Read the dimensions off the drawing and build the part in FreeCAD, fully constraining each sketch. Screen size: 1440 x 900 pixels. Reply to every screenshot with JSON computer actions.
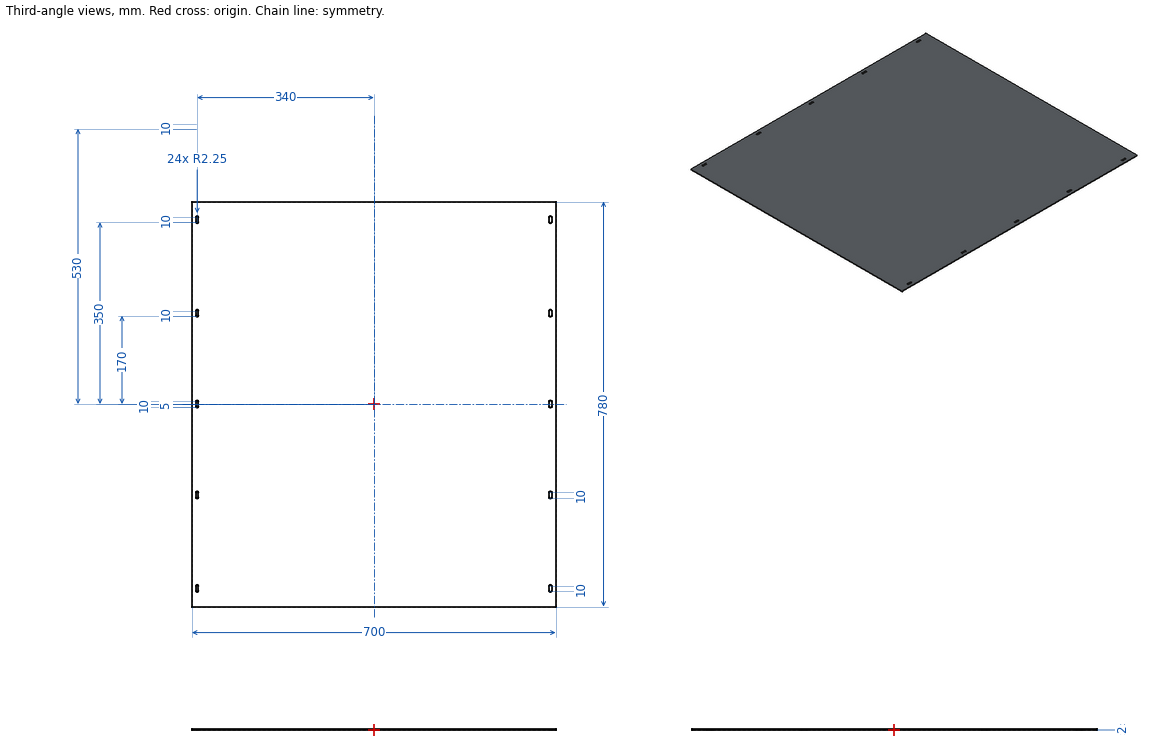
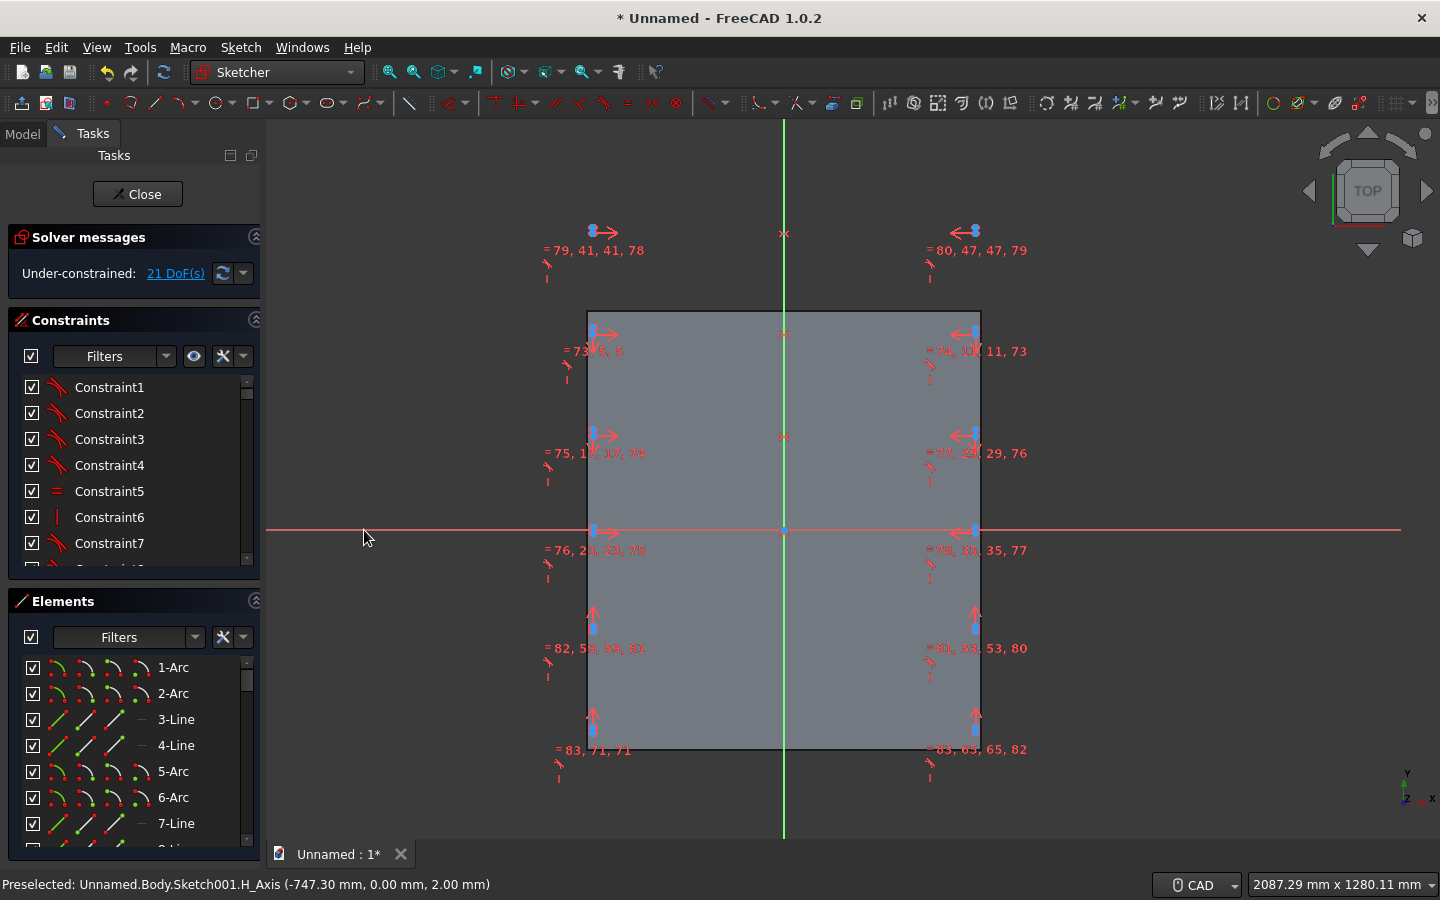
{"action": "key", "text": "d"}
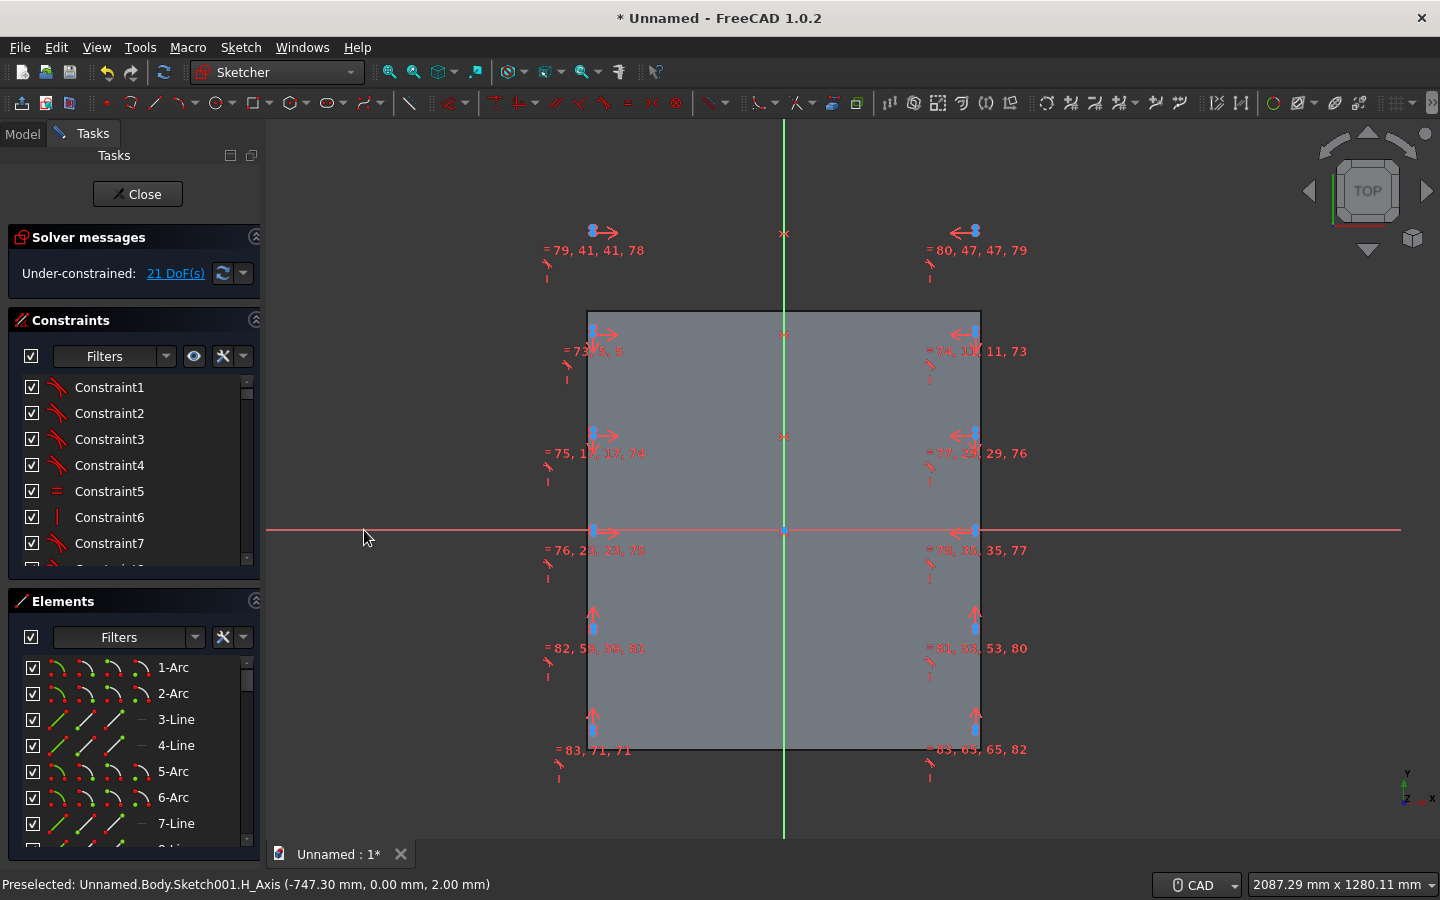
{"action": "scroll", "coordinate": [592, 331], "scroll_direction": "up", "scroll_amount": 10}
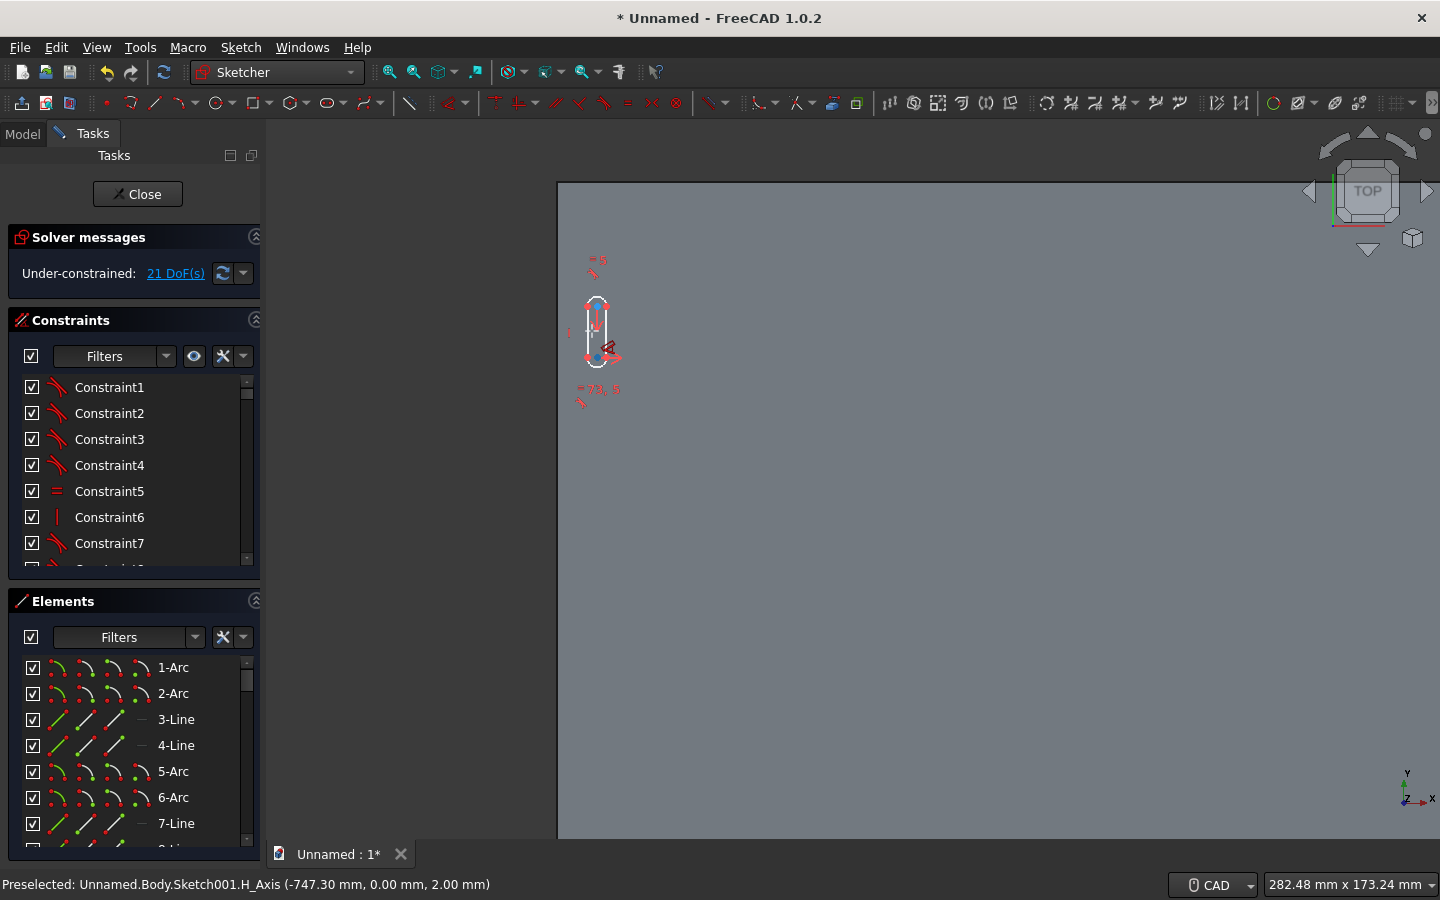
{"action": "left_click", "coordinate": [588, 327]}
{"action": "left_click", "coordinate": [554, 332]}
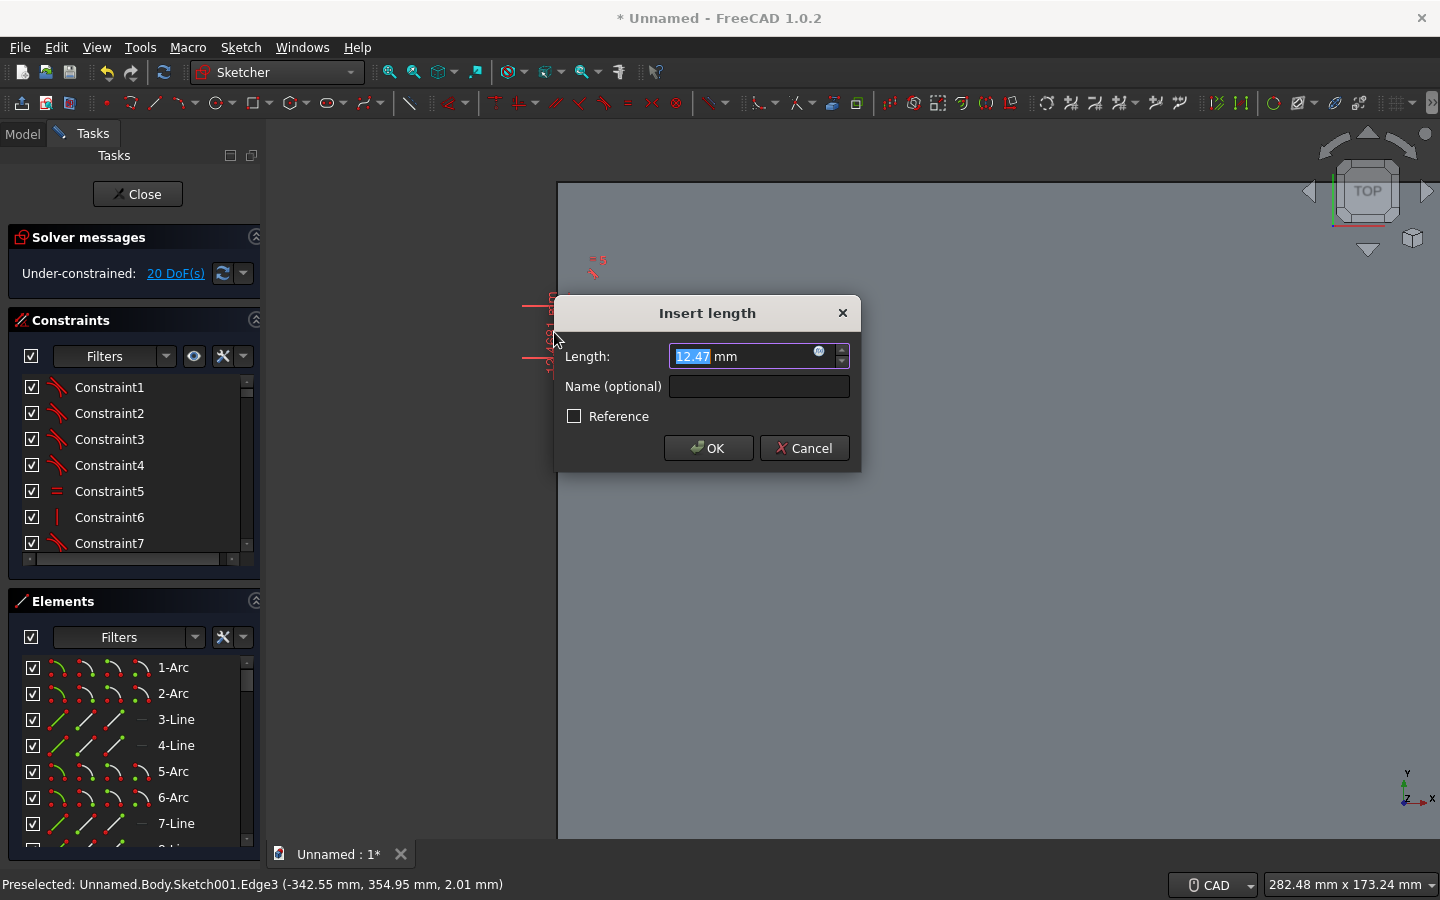
{"action": "type", "text": "10"}
{"action": "key", "text": "Return"}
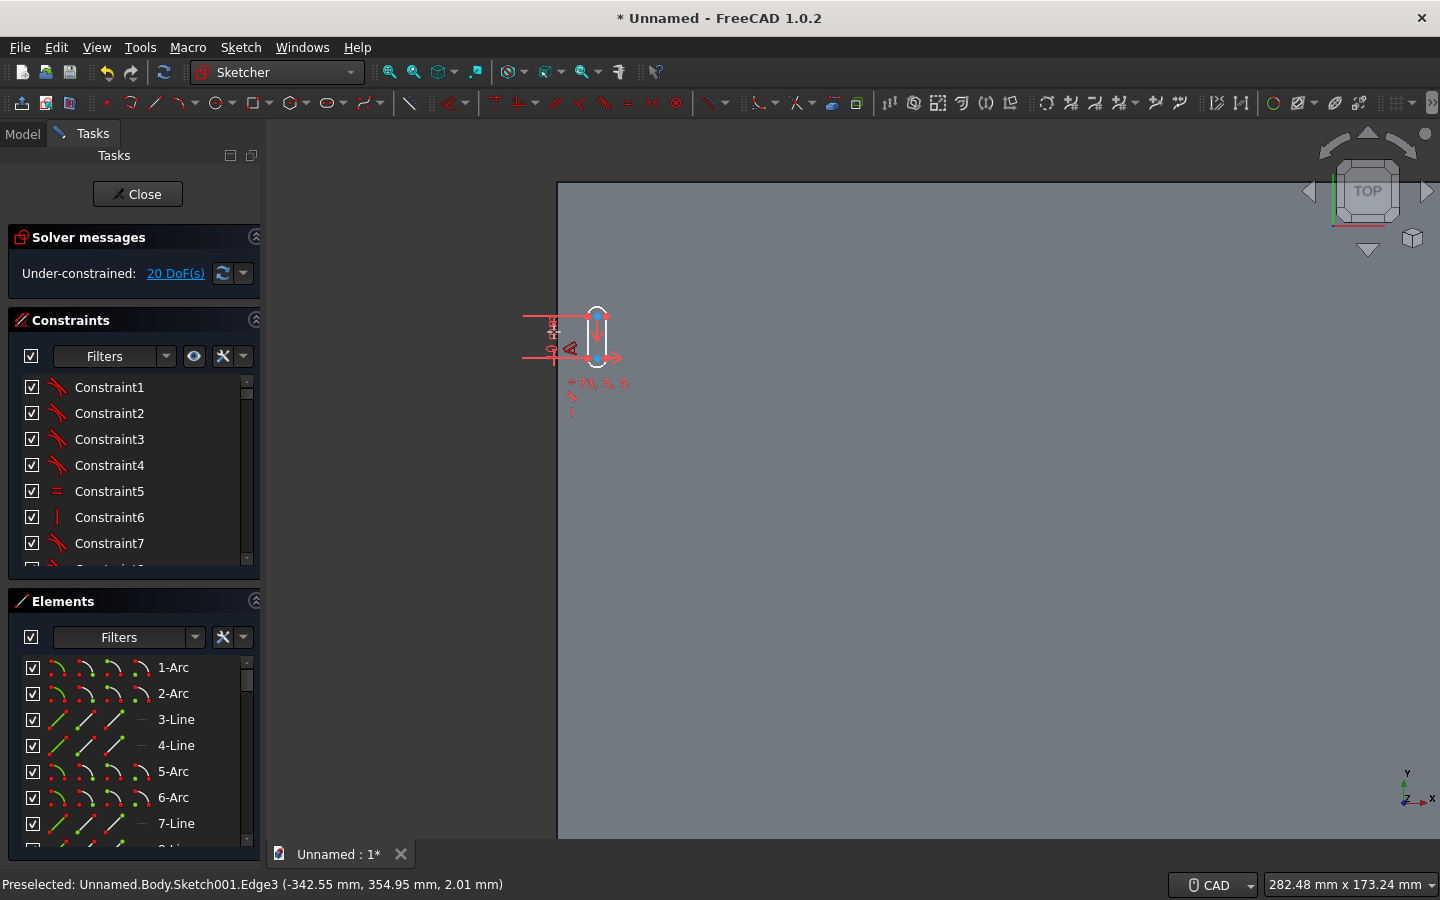
{"action": "scroll", "coordinate": [592, 330], "scroll_direction": "down", "scroll_amount": 10}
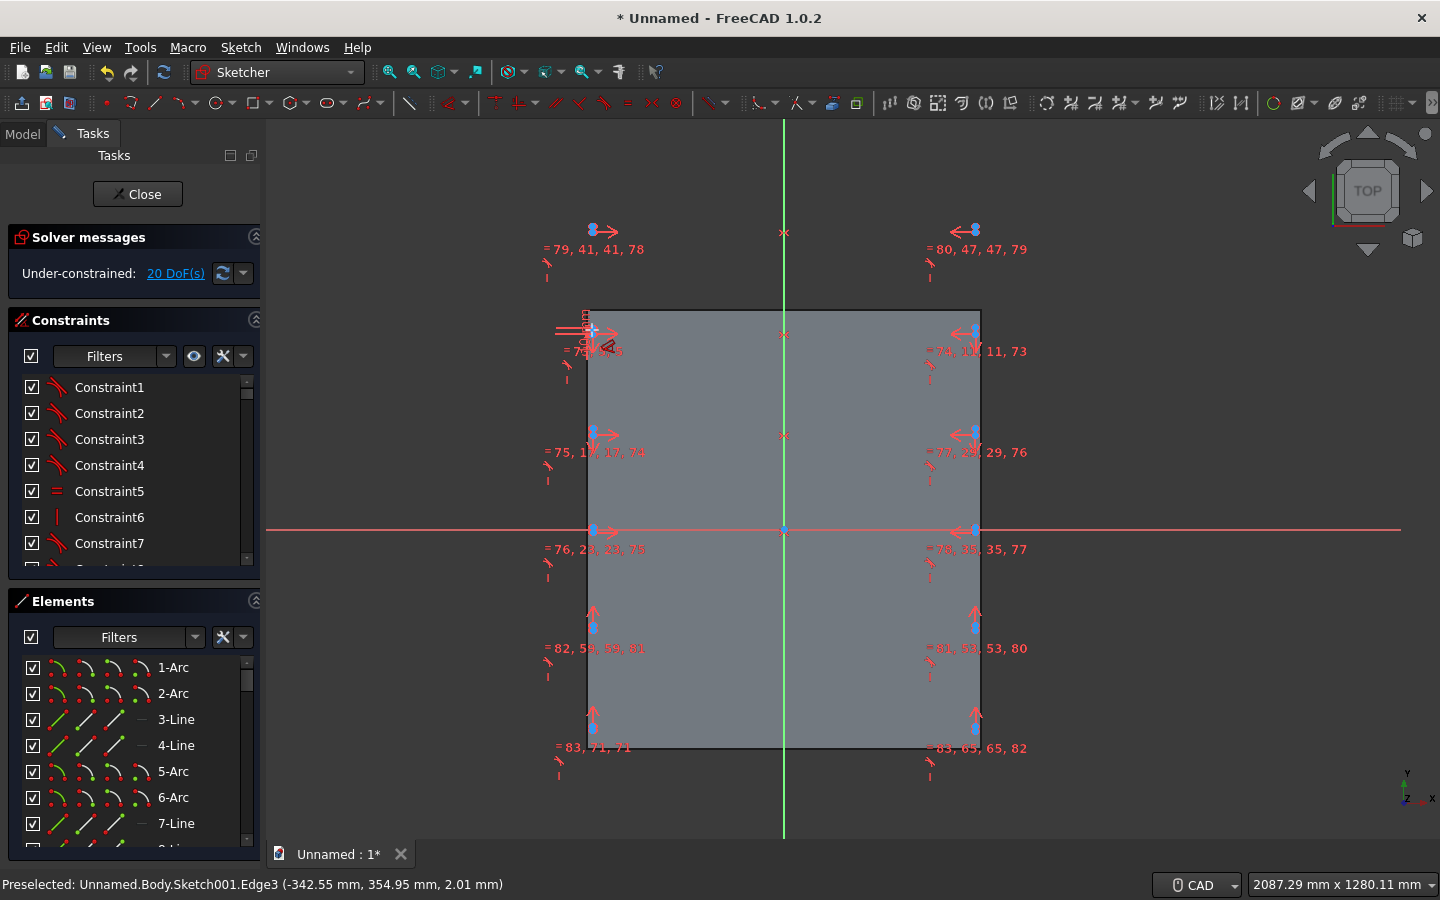
{"action": "scroll", "coordinate": [974, 332], "scroll_direction": "up", "scroll_amount": 10}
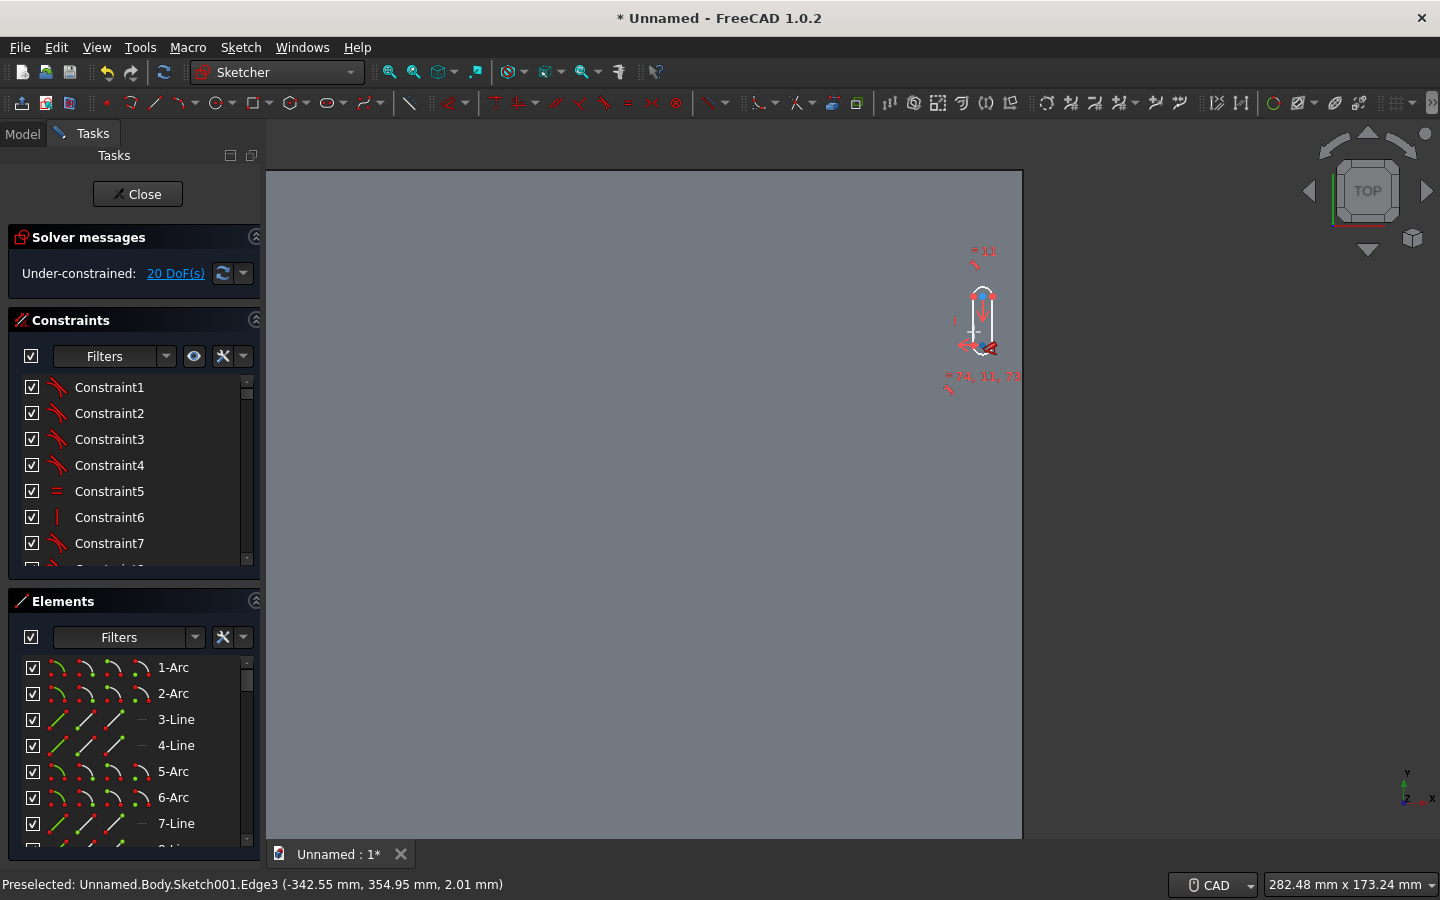
{"action": "left_click", "coordinate": [973, 331]}
{"action": "left_click", "coordinate": [1007, 321]}